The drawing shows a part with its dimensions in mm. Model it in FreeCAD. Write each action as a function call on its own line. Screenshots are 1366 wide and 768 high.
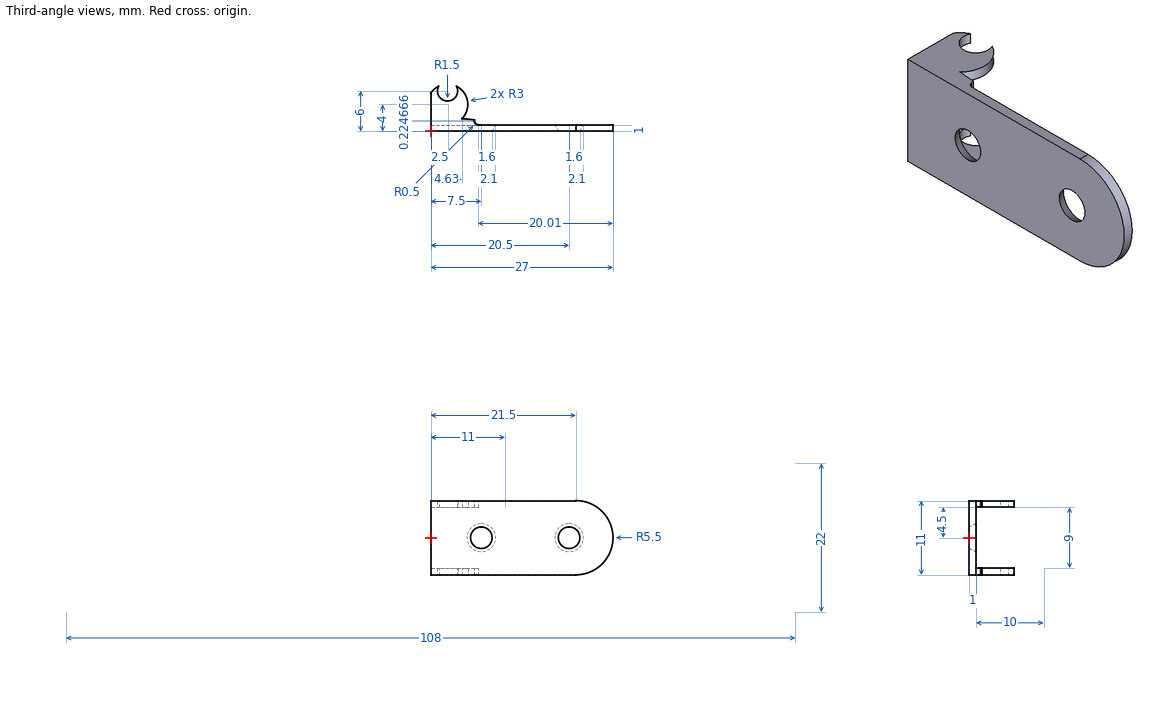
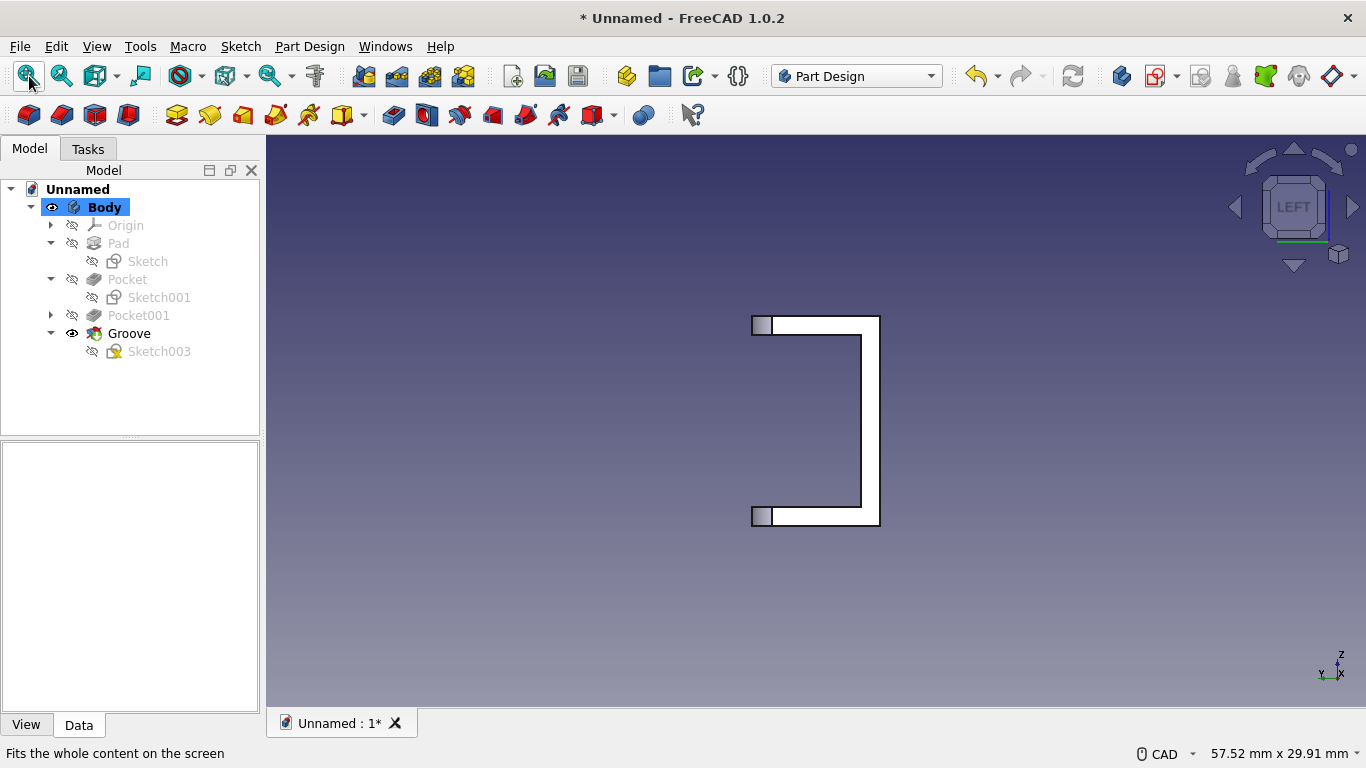
click(1154, 76)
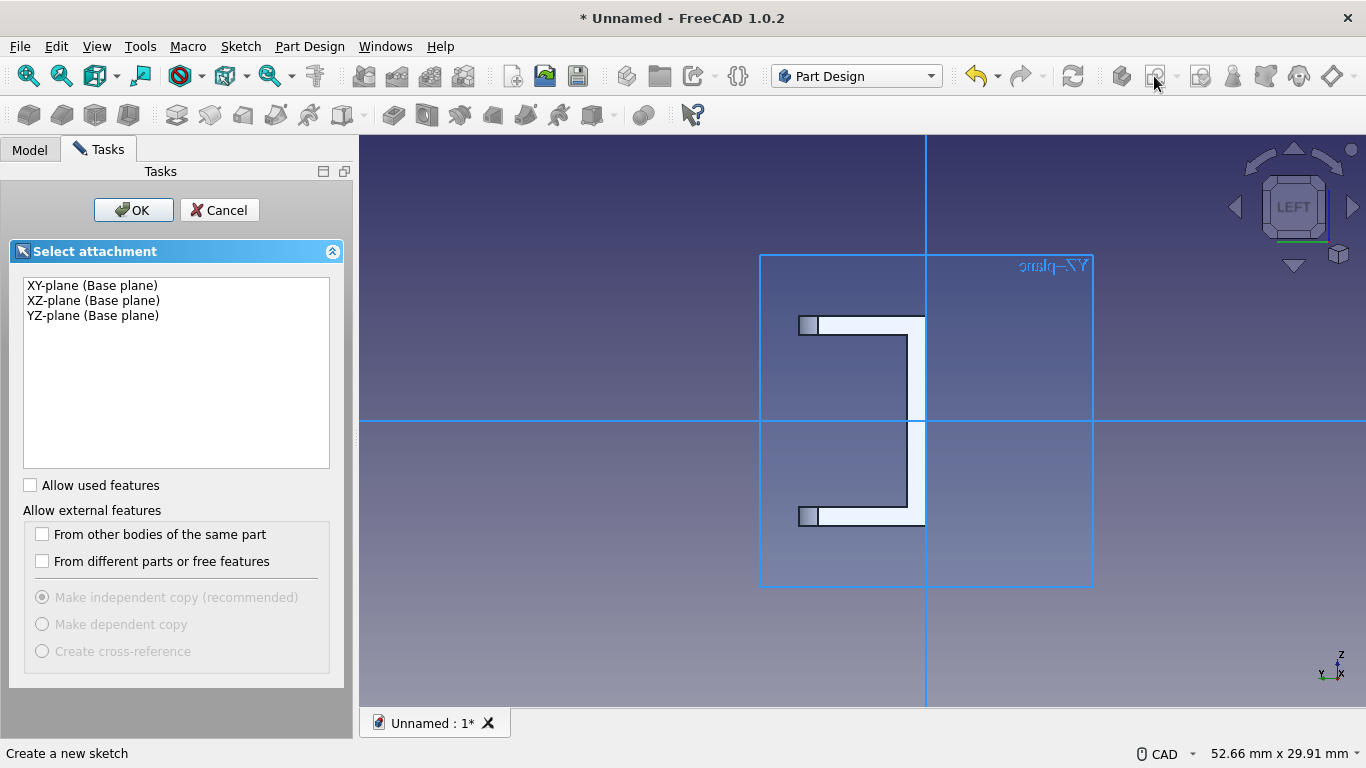
click(84, 286)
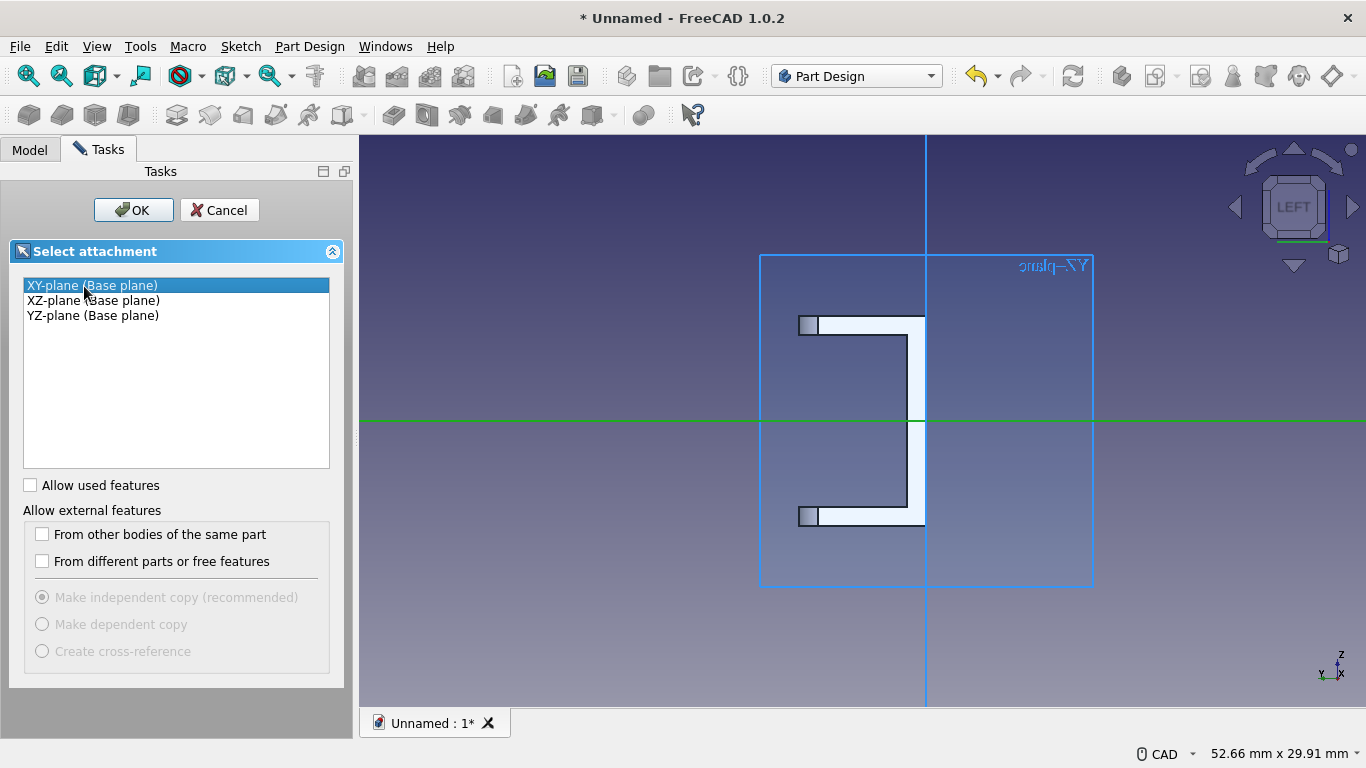
click(134, 210)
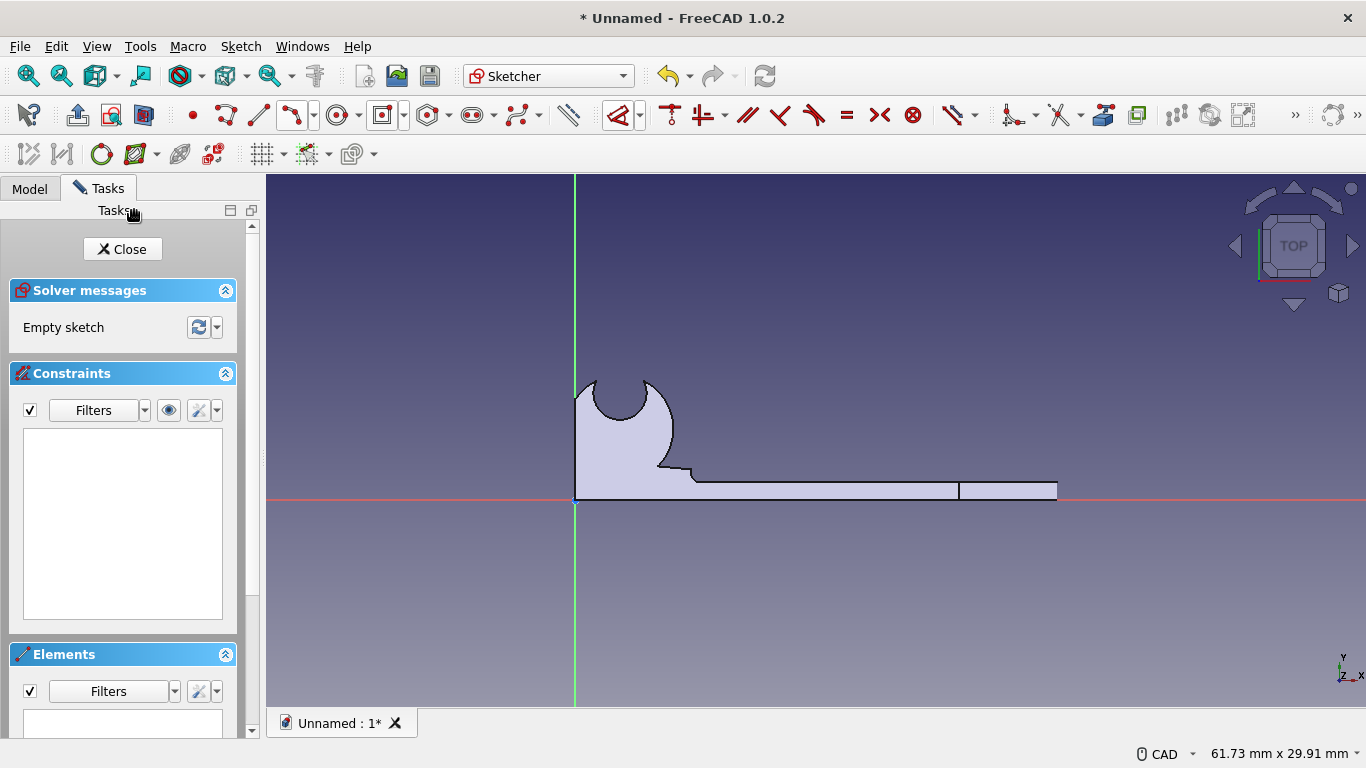
click(144, 116)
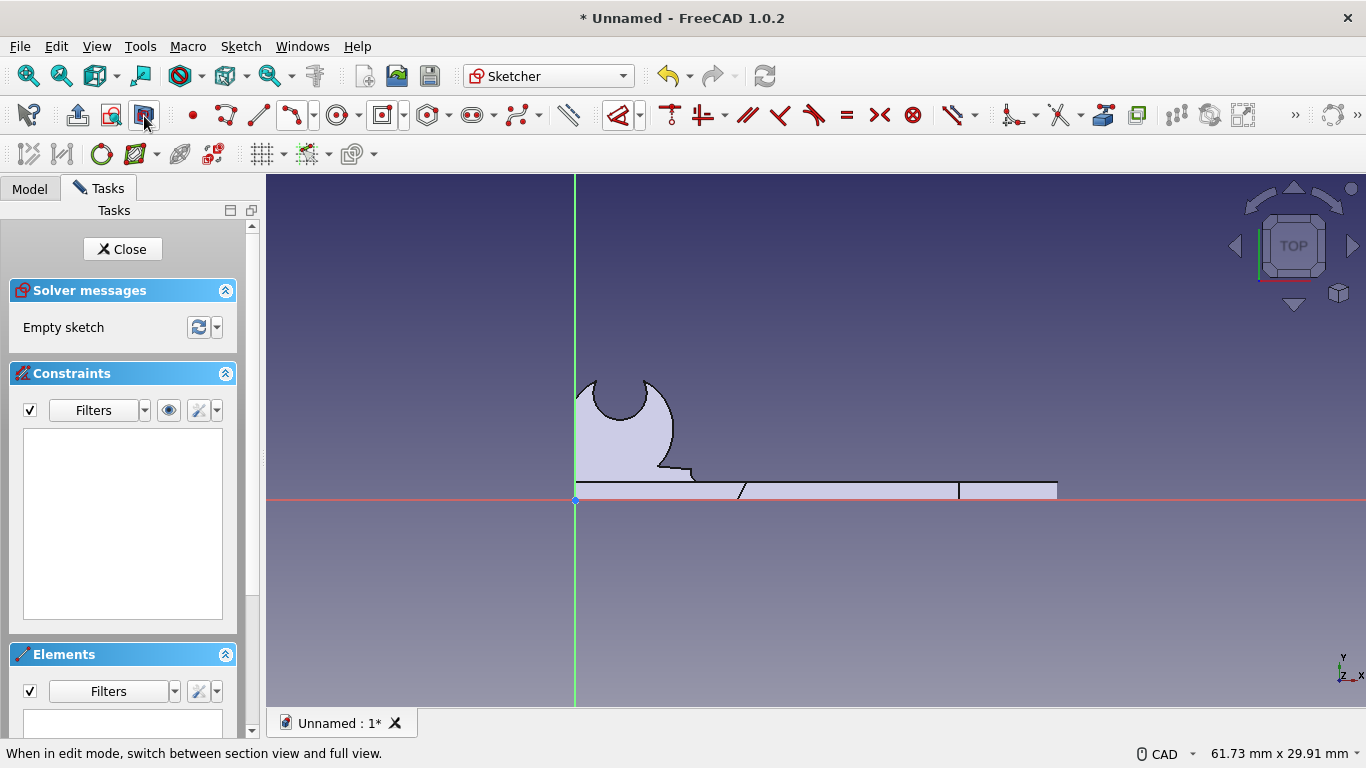
scroll(976, 491, up, 13)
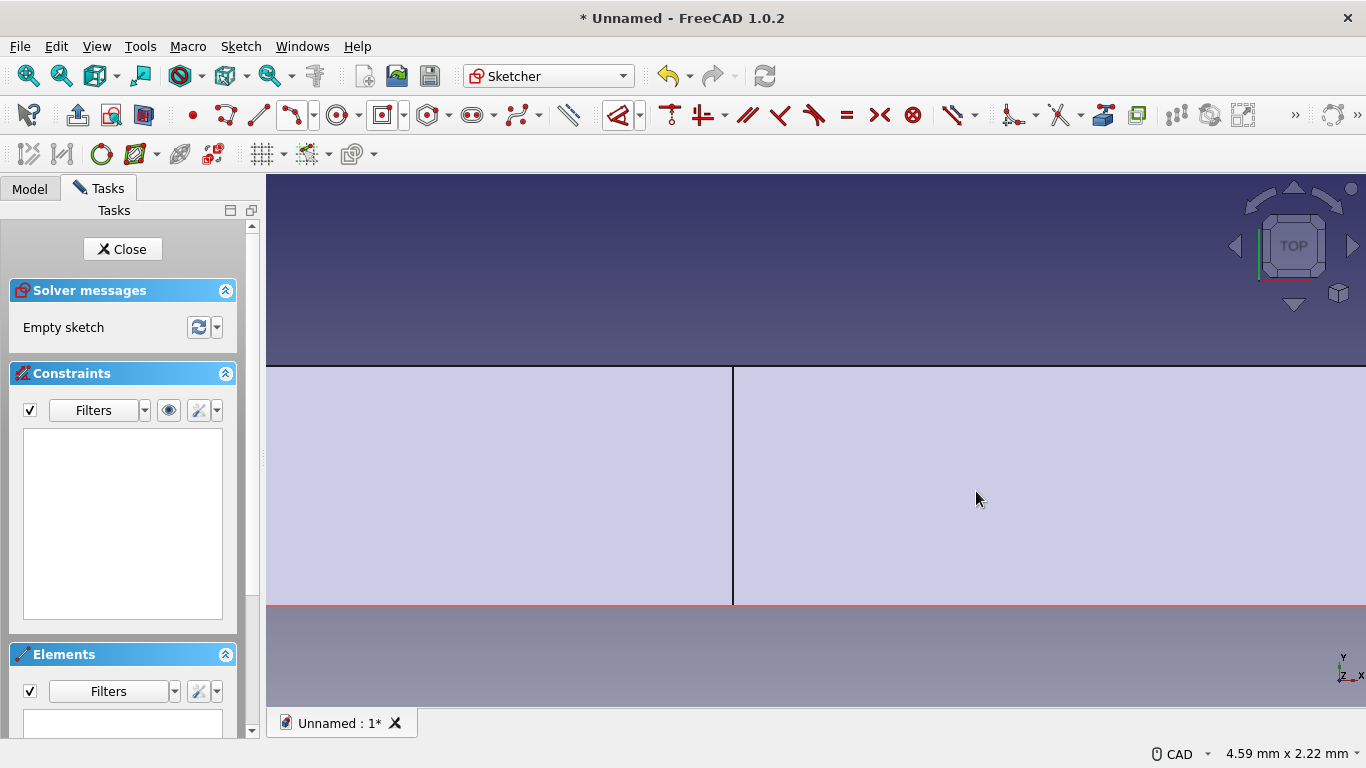
key(g)
key(m)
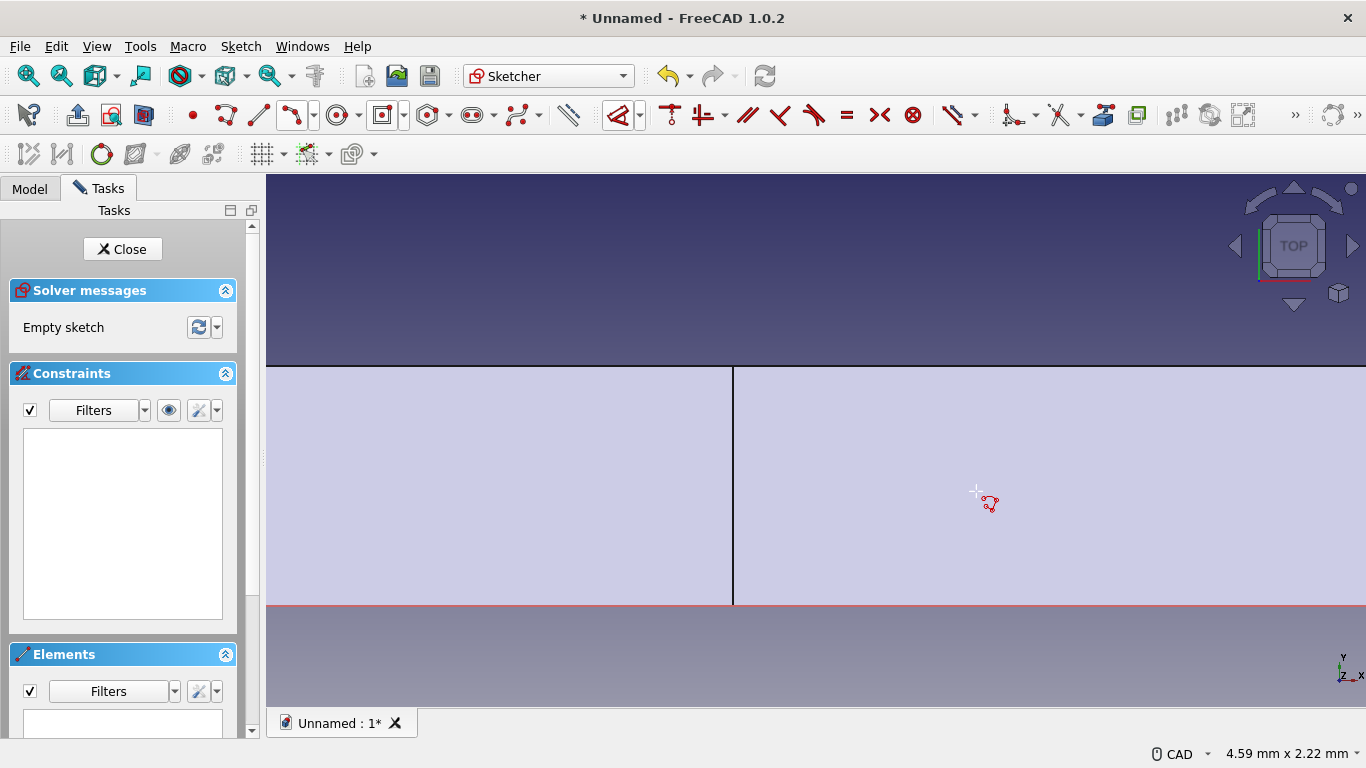
click(493, 606)
click(877, 597)
click(997, 366)
click(493, 366)
click(493, 606)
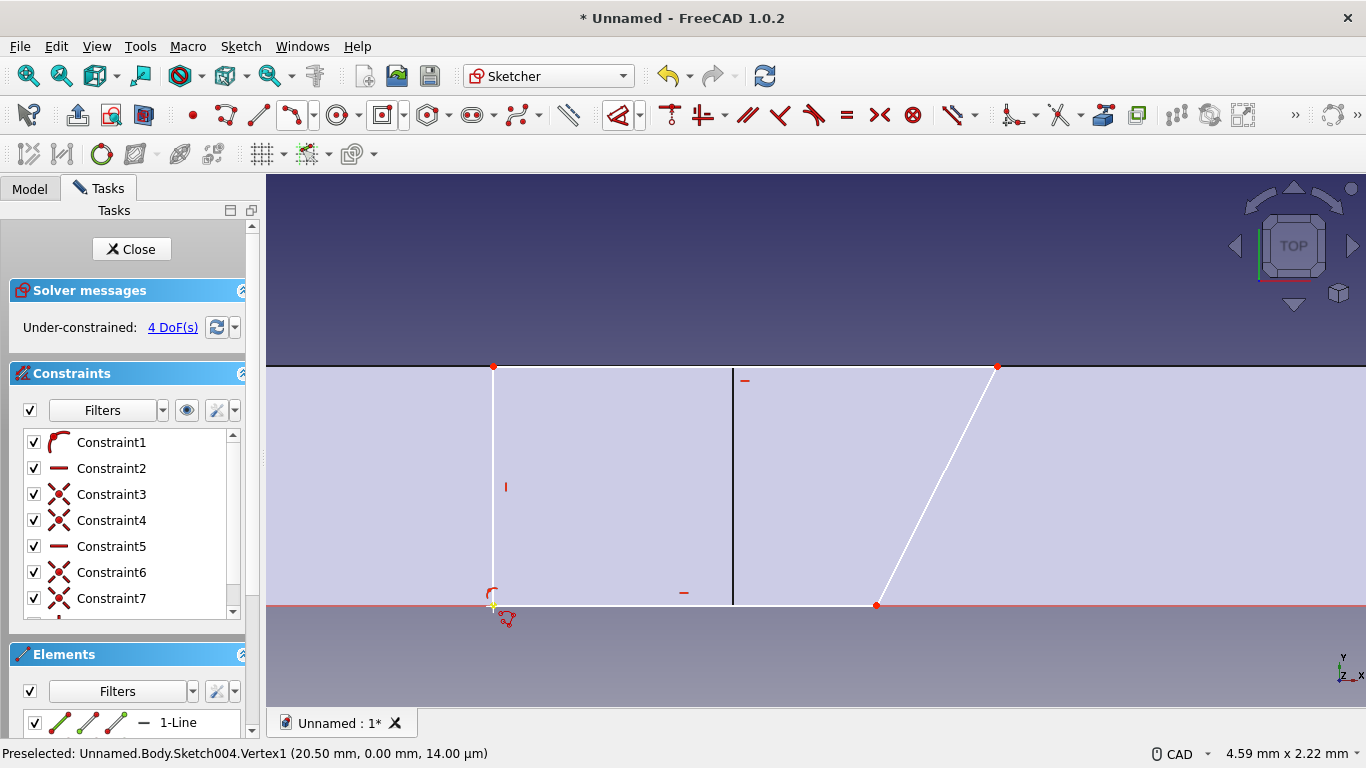
key(g)
key(l)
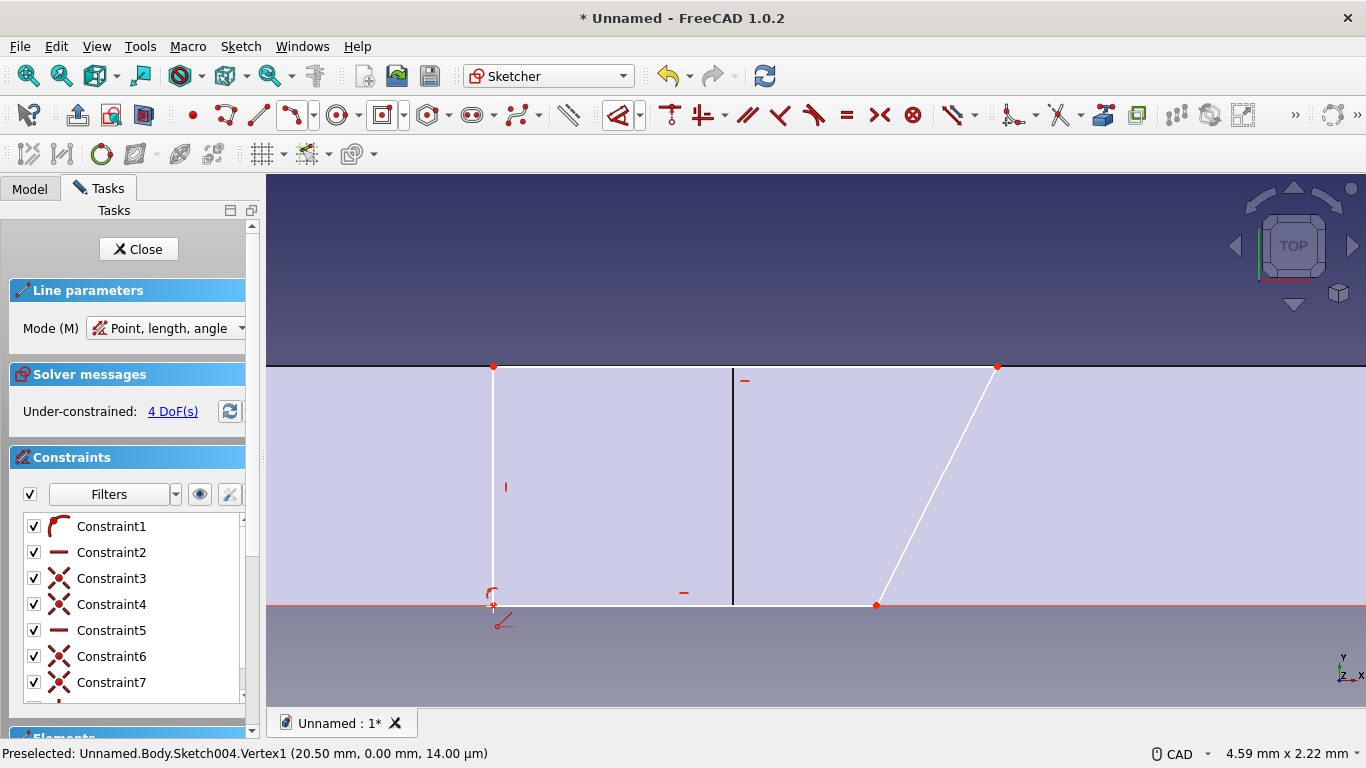
click(493, 342)
click(493, 270)
key(Escape)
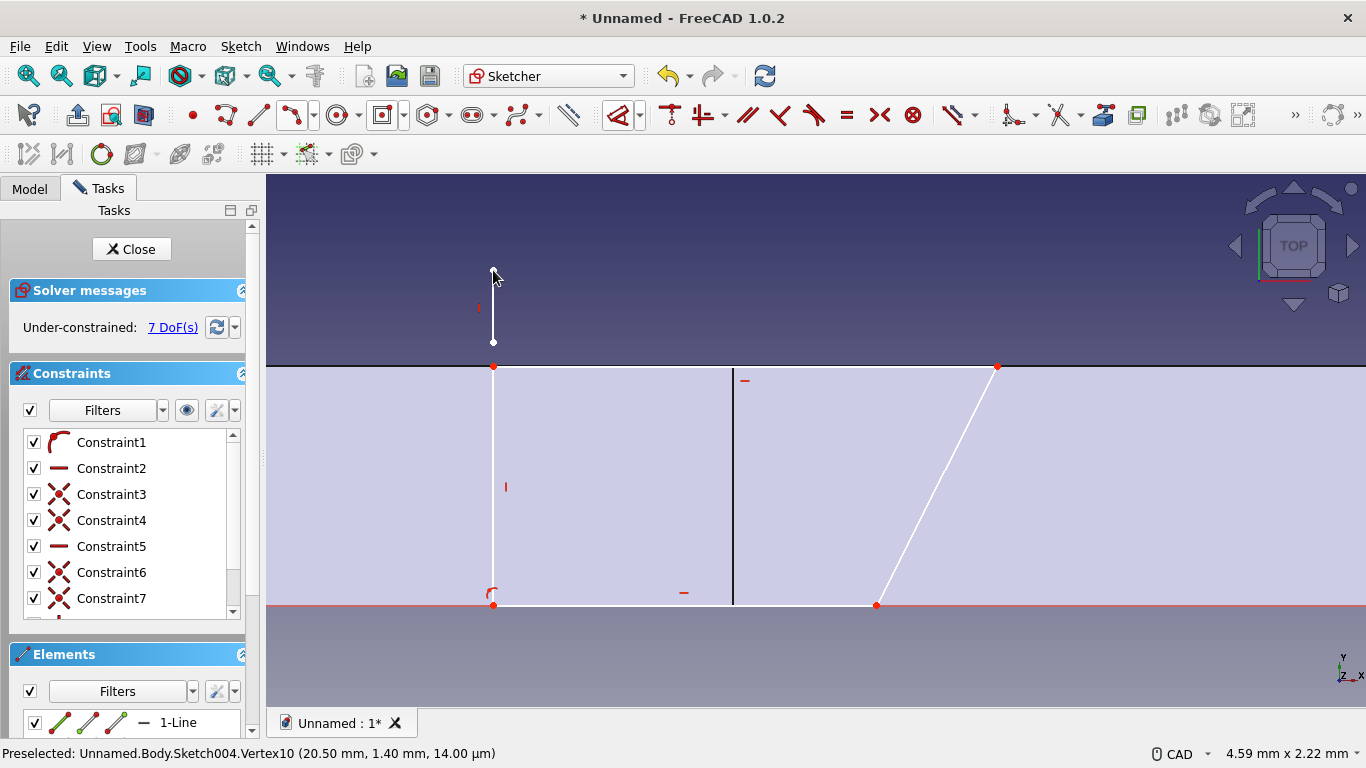
click(493, 321)